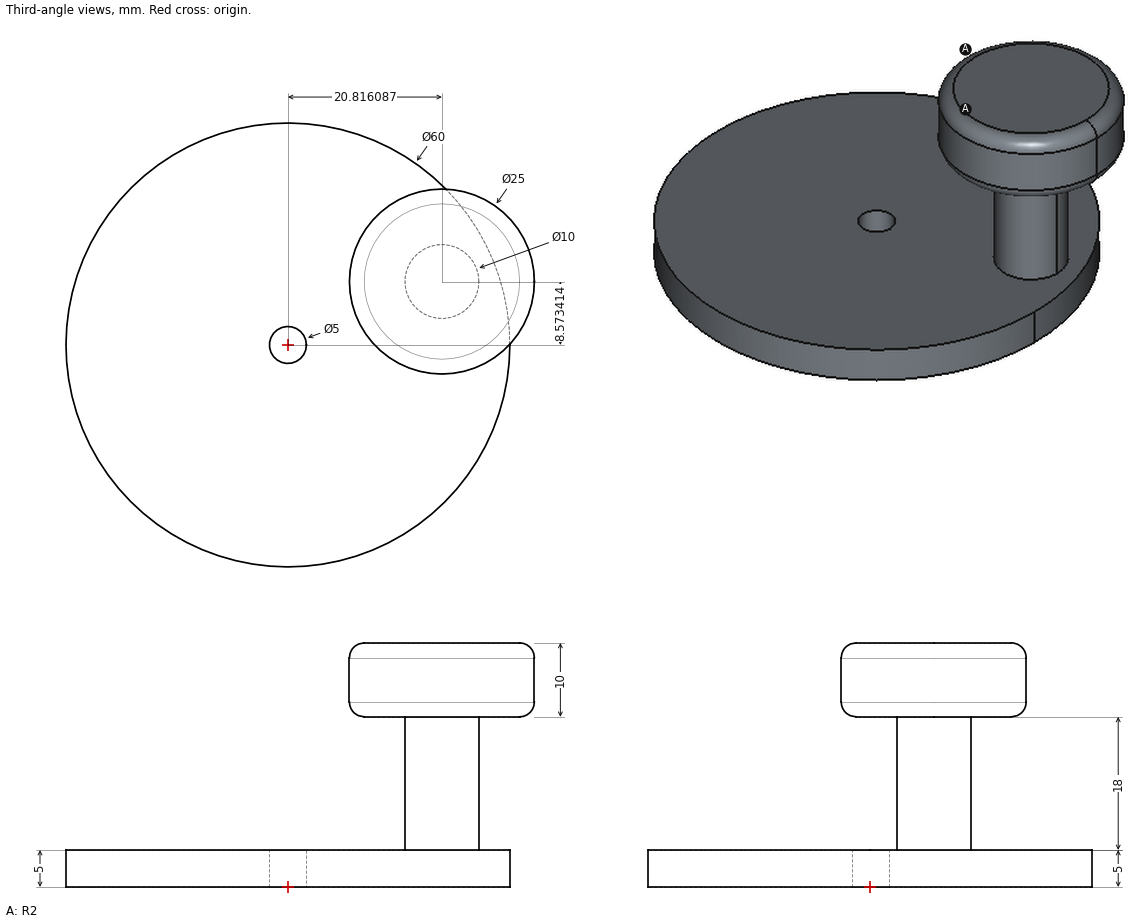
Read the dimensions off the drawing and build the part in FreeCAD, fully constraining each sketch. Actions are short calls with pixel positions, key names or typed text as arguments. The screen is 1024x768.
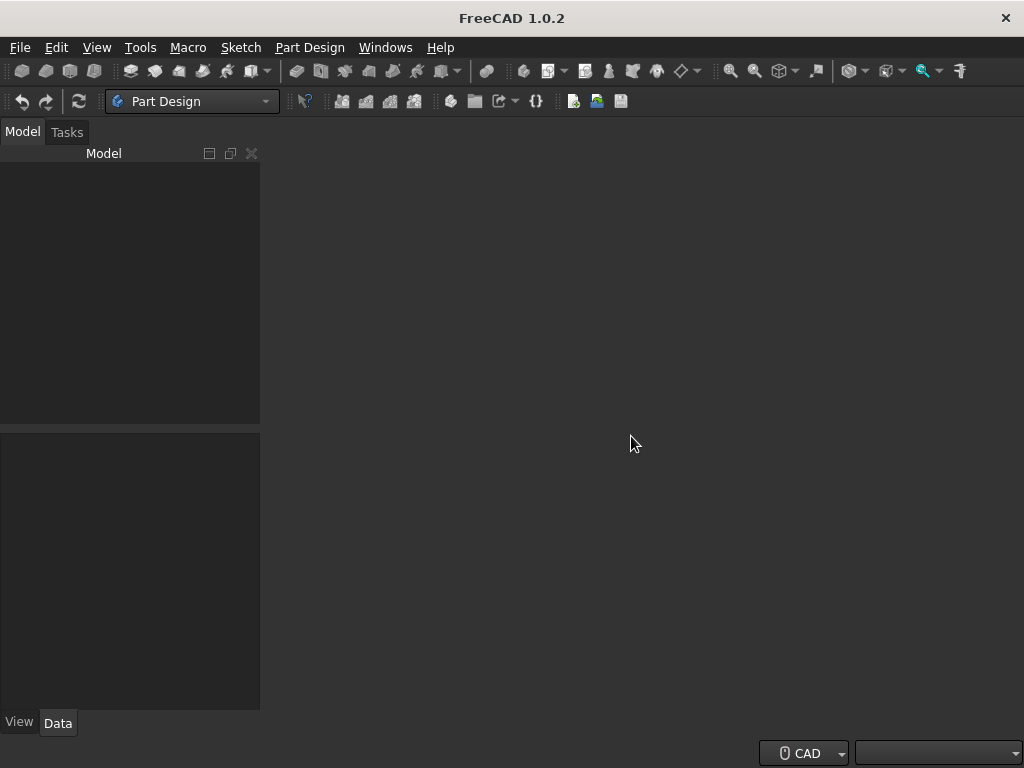
click(574, 102)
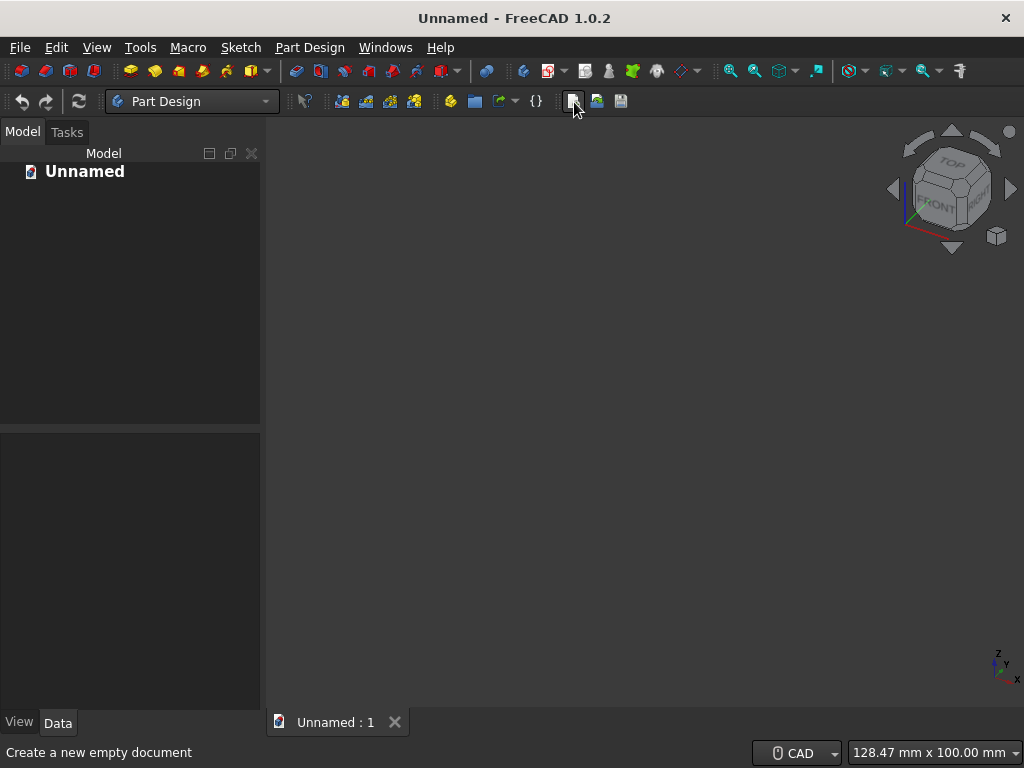
click(548, 72)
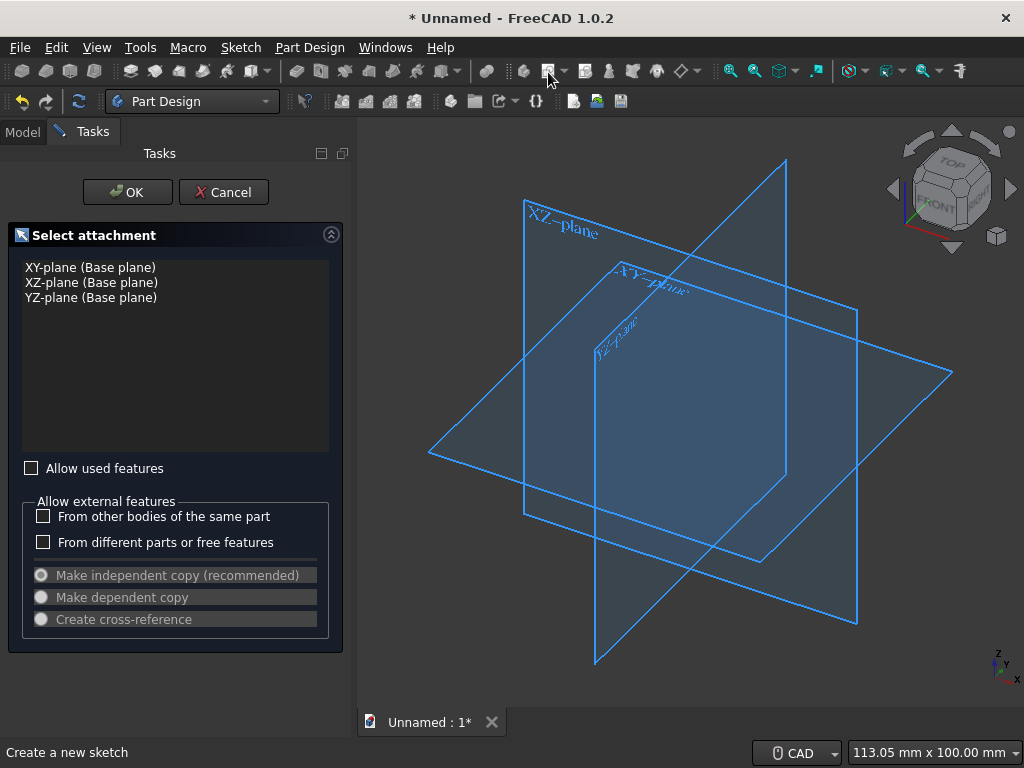
click(82, 268)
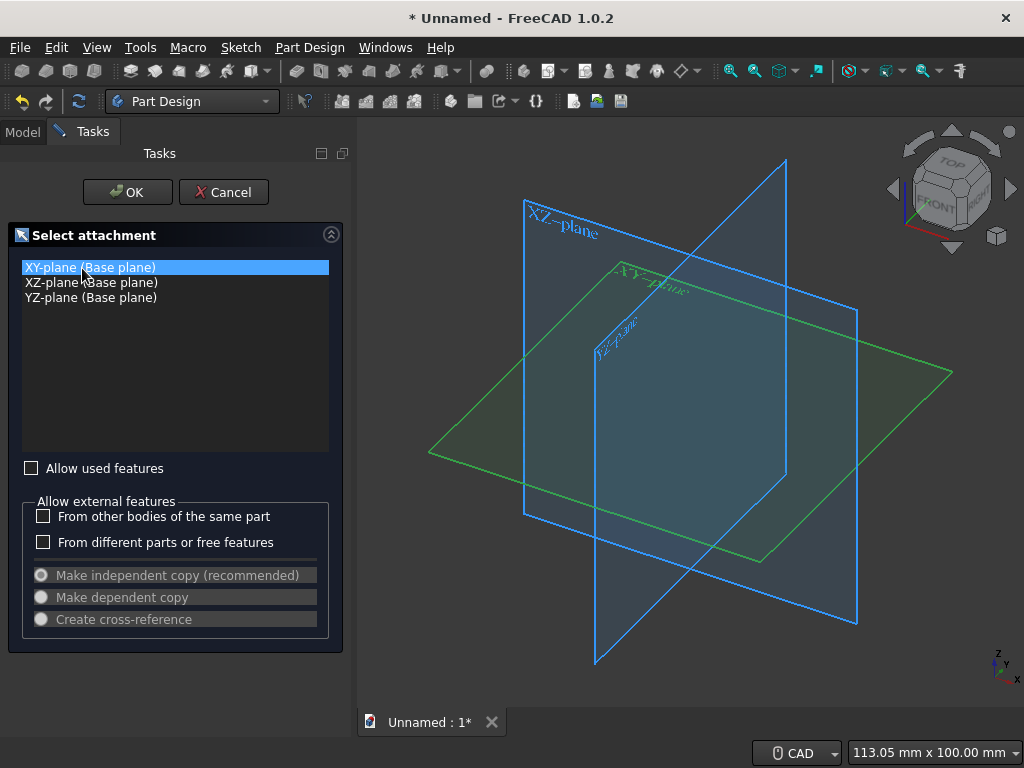
click(128, 192)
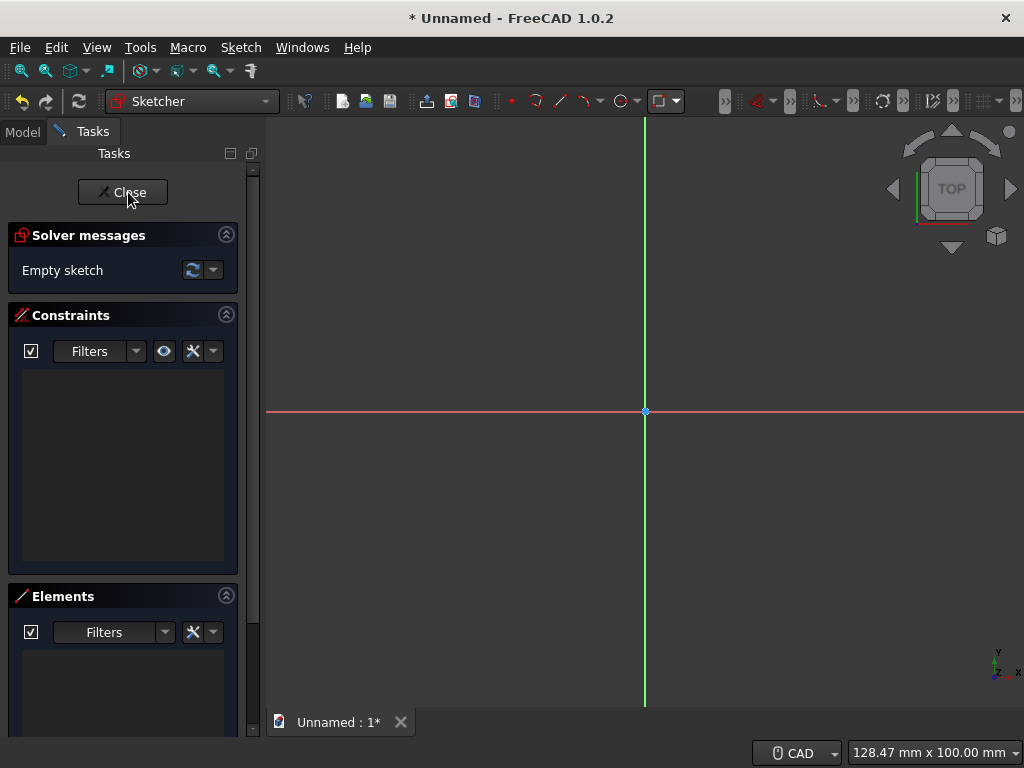
click(622, 102)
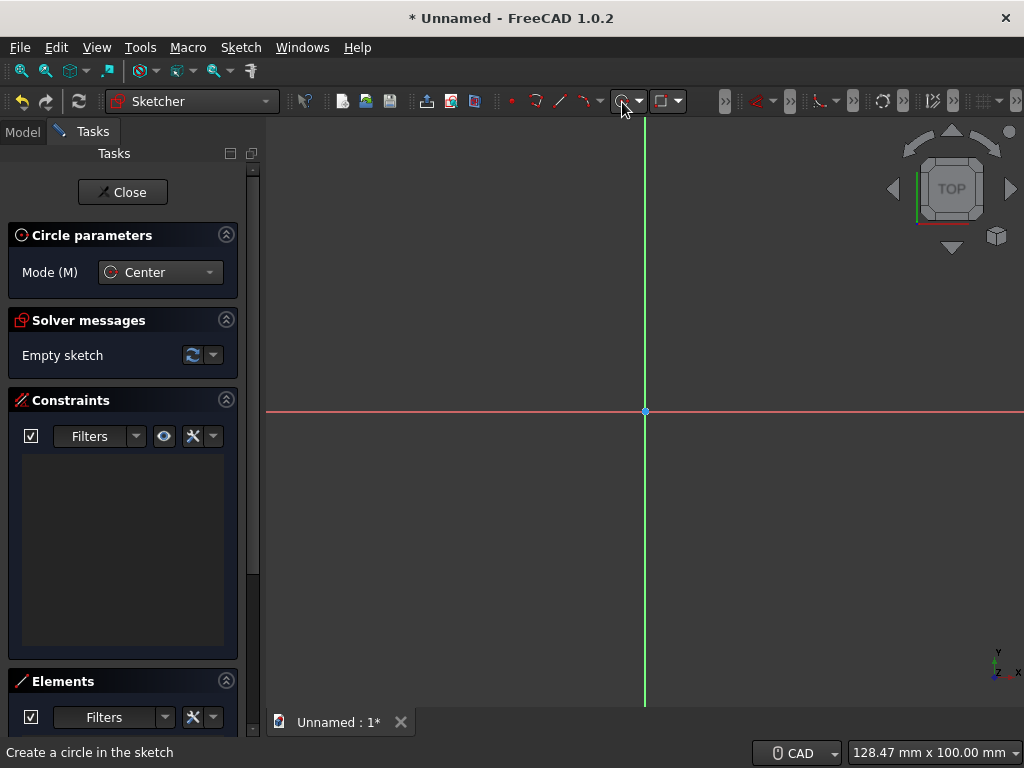
click(645, 412)
move(770, 287)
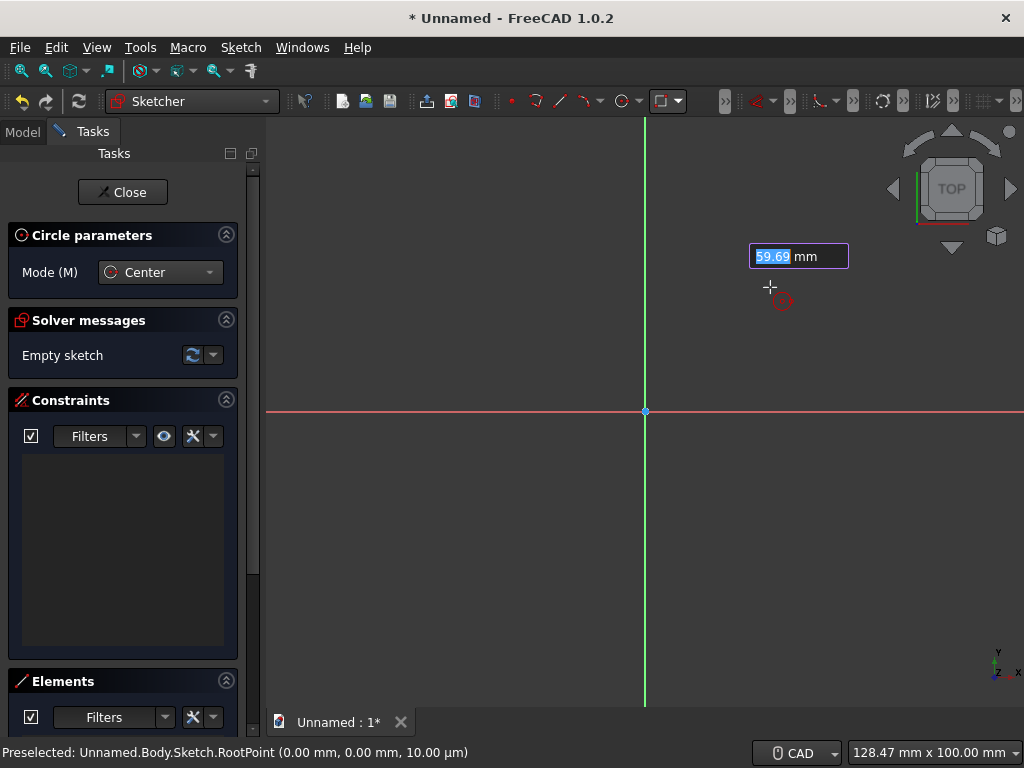
text(60)
key(Return)
key(Escape)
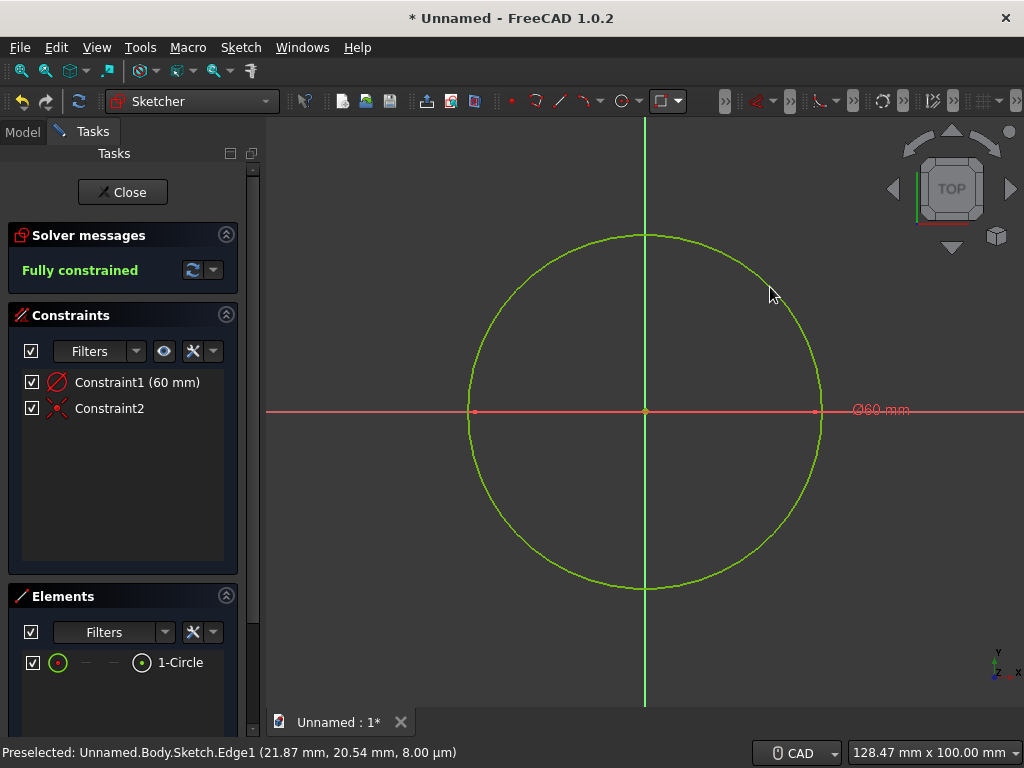
click(123, 192)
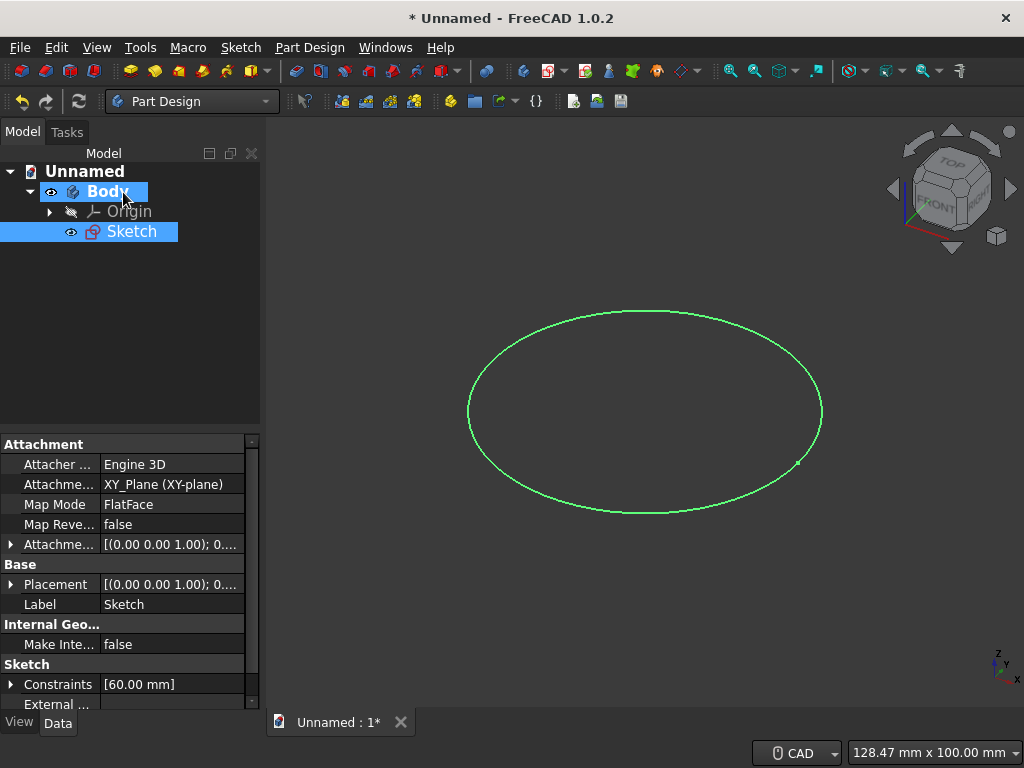
click(132, 72)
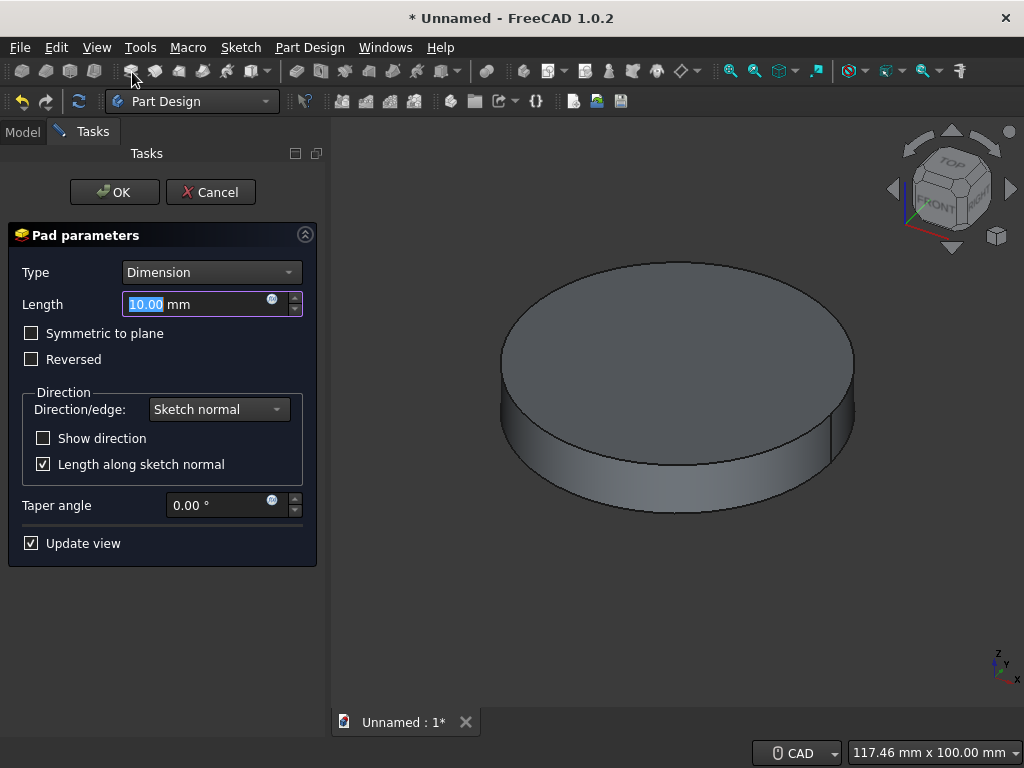
text(5)
key(Tab)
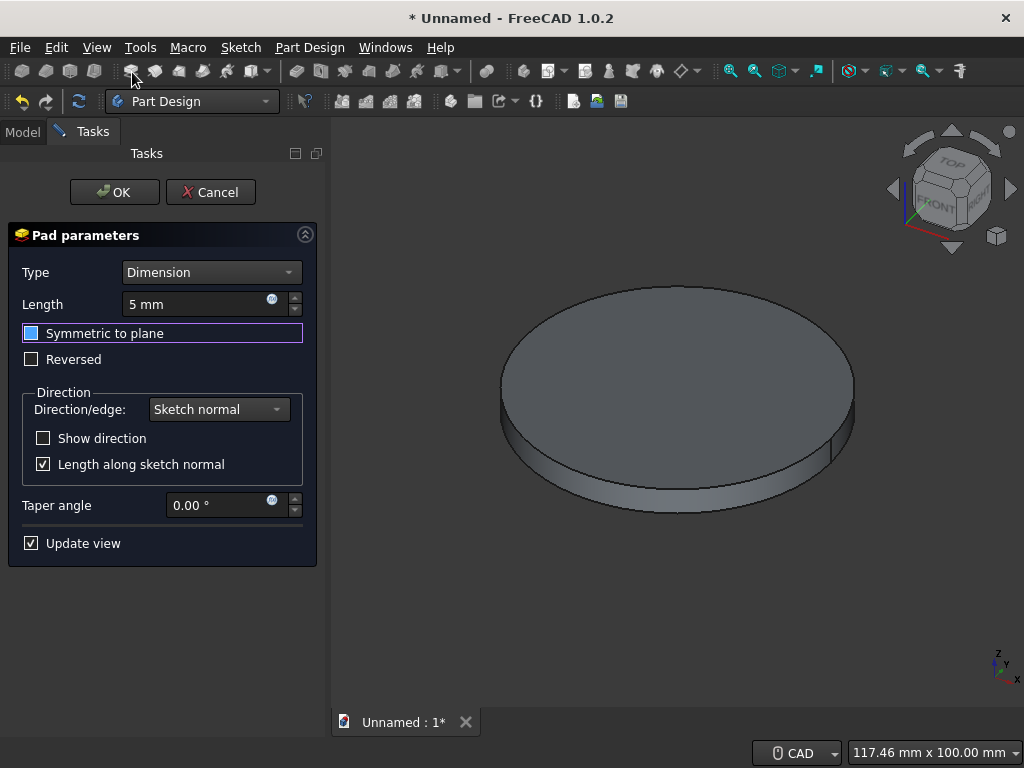
click(115, 192)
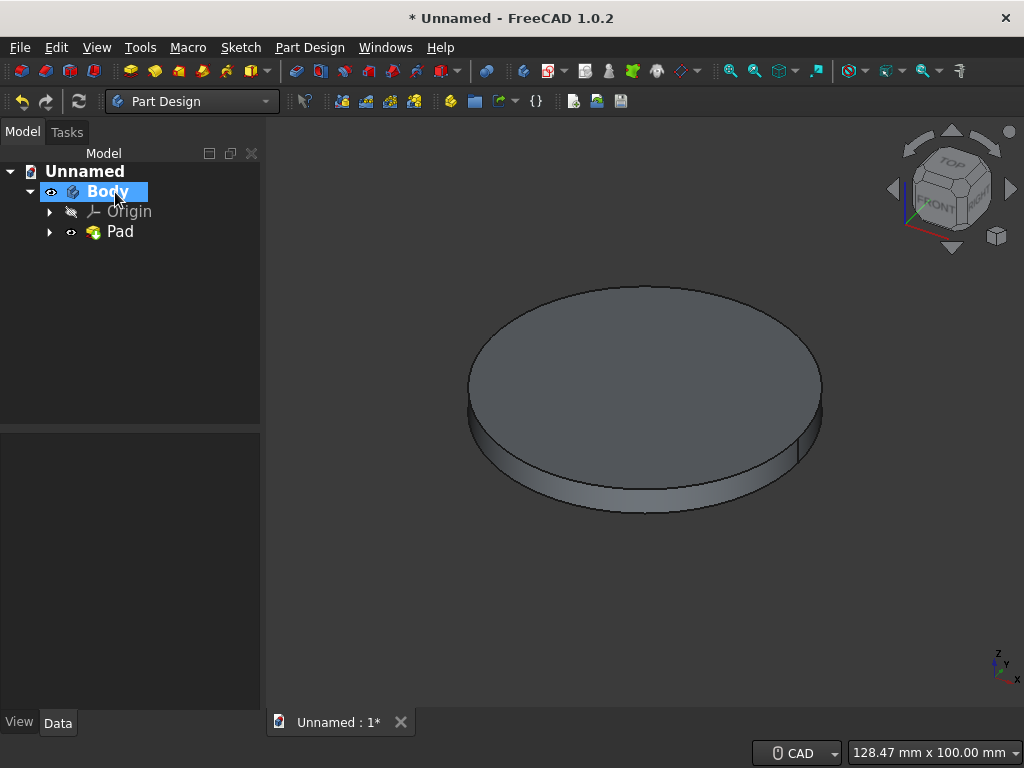
click(645, 387)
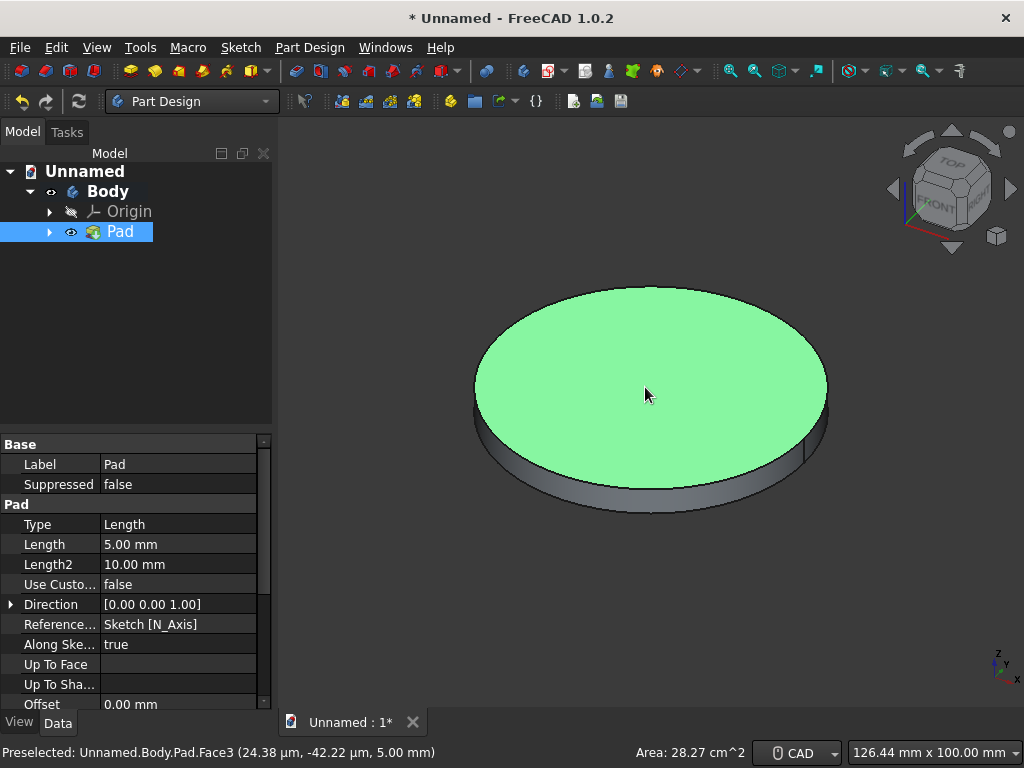
click(548, 72)